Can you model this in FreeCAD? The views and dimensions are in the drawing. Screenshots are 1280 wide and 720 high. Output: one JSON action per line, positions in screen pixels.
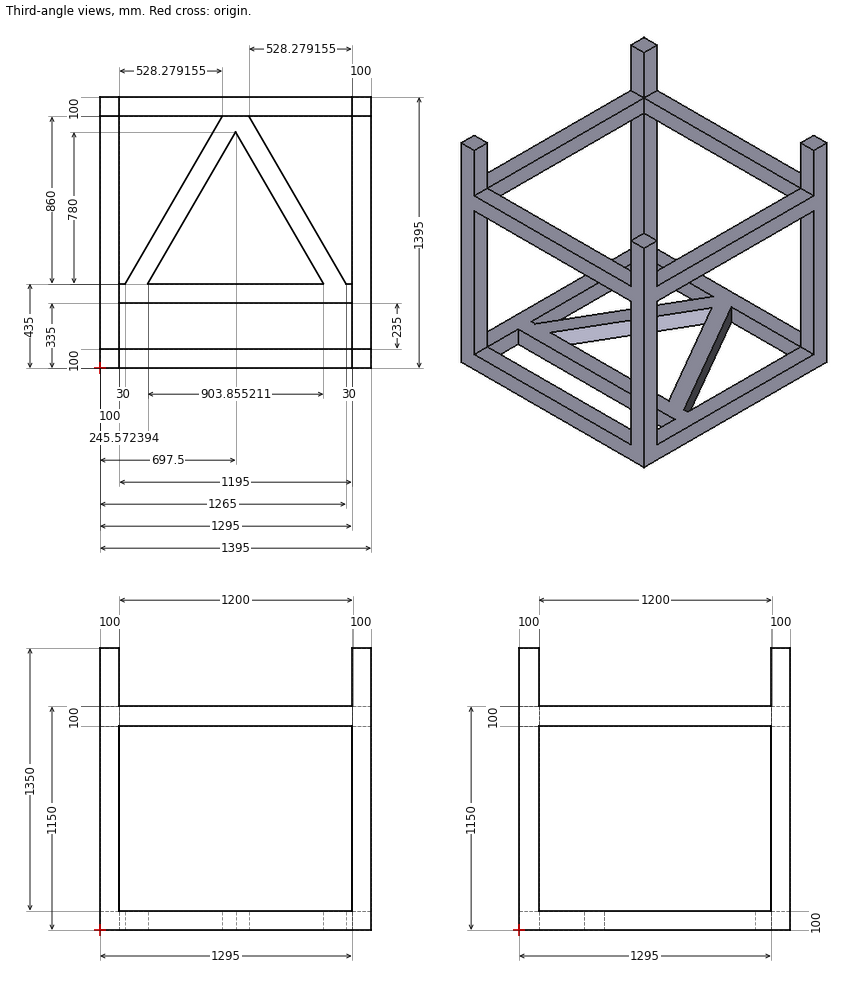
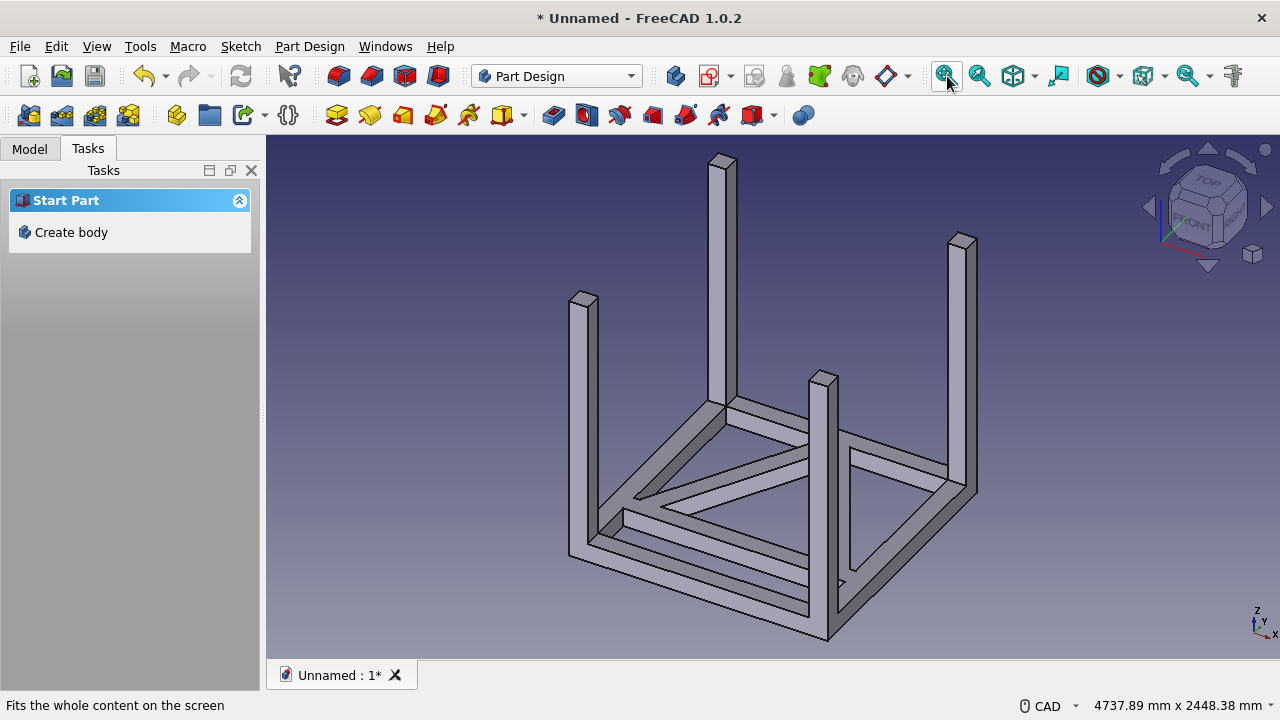
{"action": "left_click", "coordinate": [30, 148]}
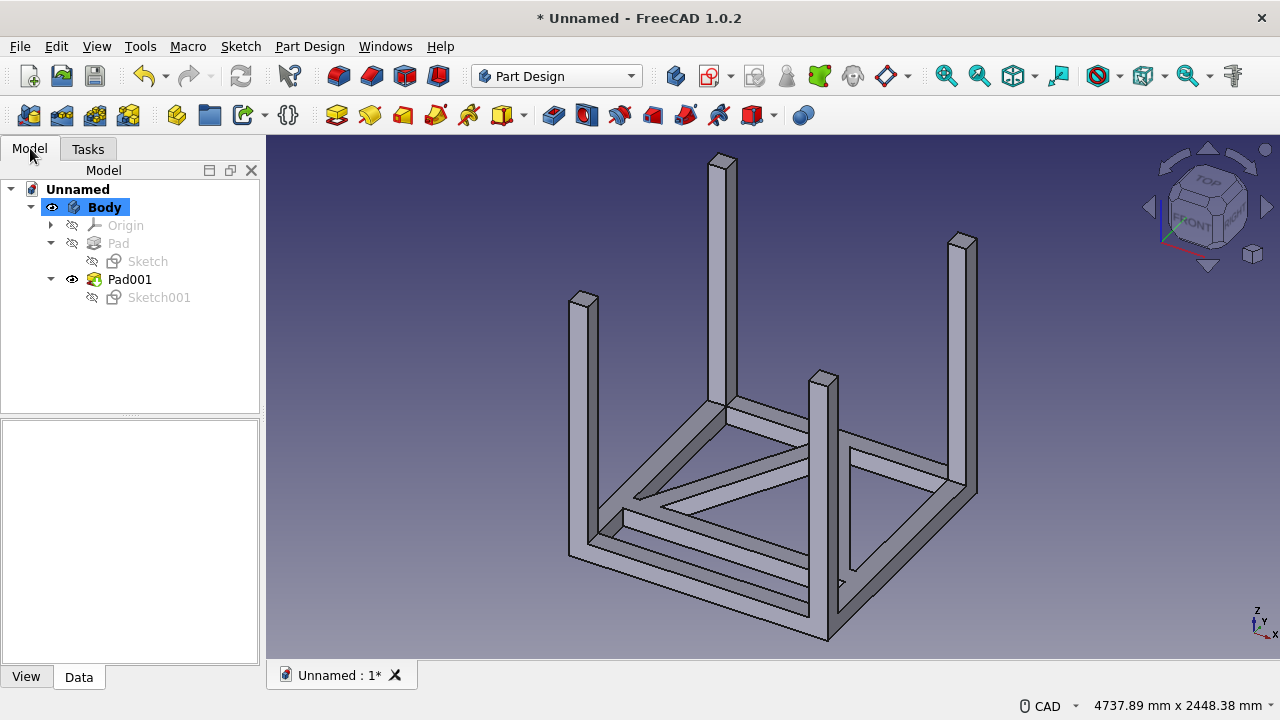
{"action": "left_click", "coordinate": [51, 225]}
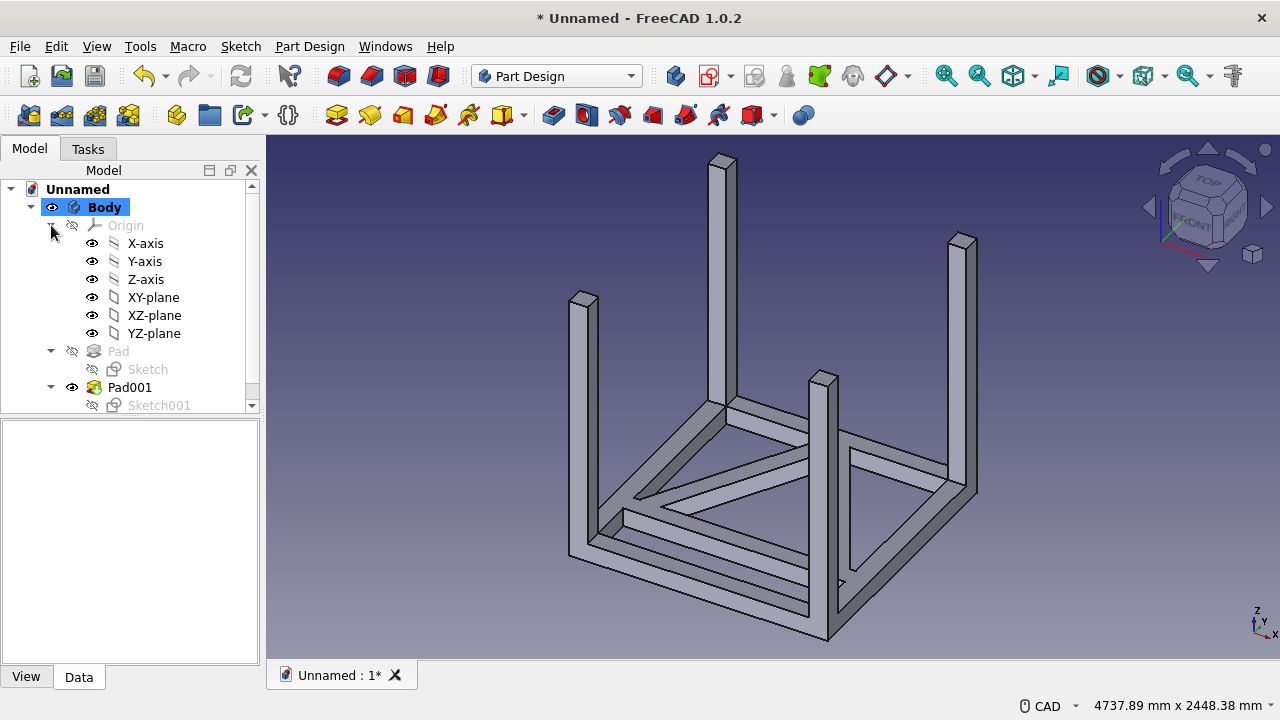
{"action": "left_click", "coordinate": [137, 333]}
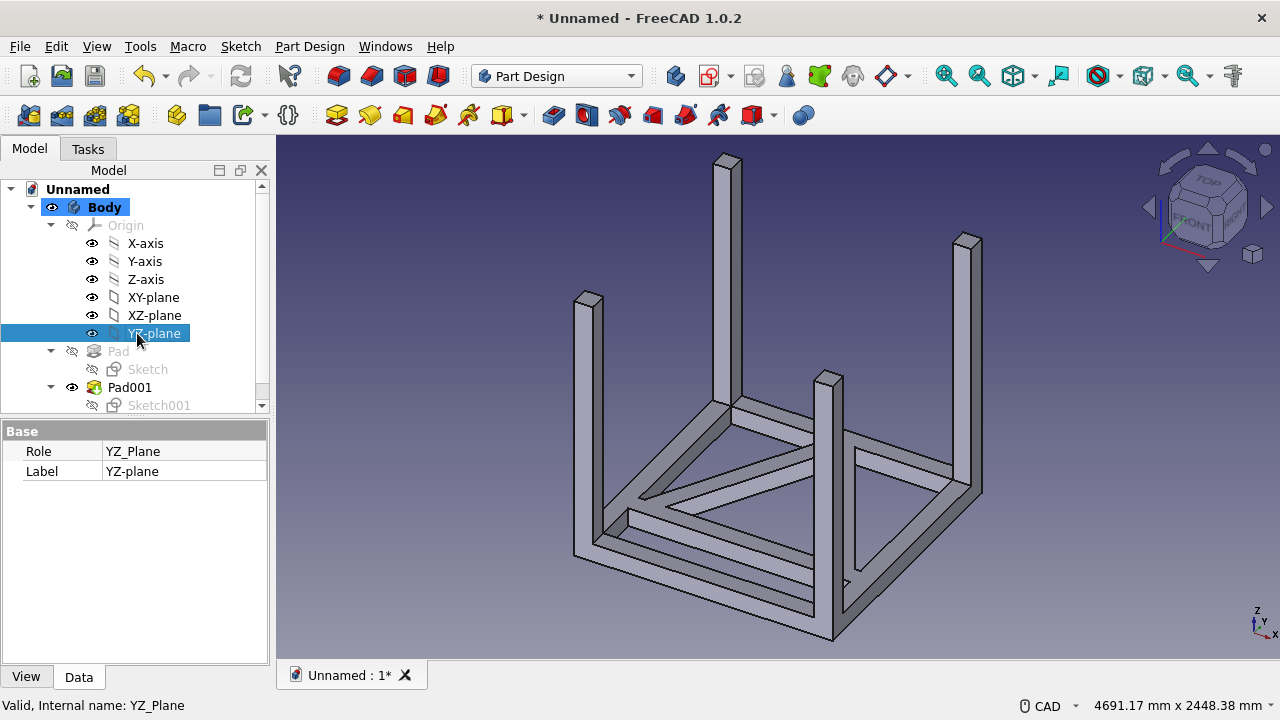
{"action": "left_click", "coordinate": [886, 76]}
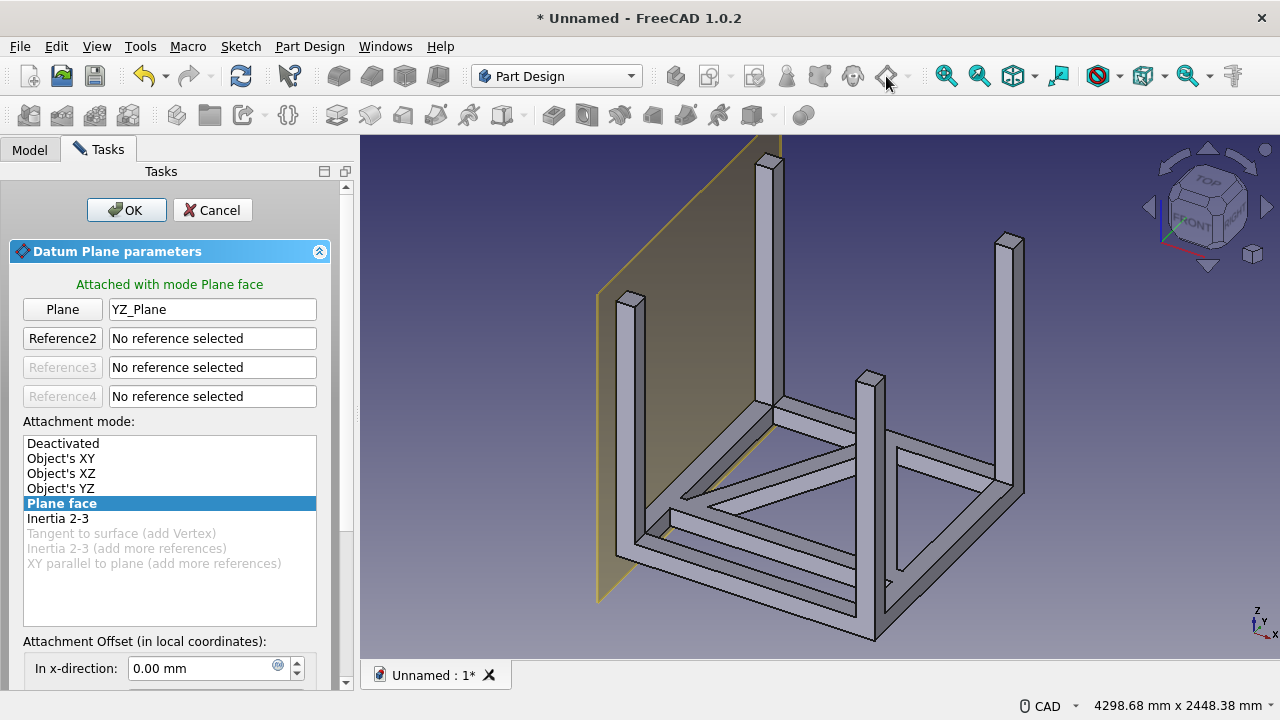
{"action": "scroll", "coordinate": [346, 436], "scroll_direction": "down", "scroll_amount": 2}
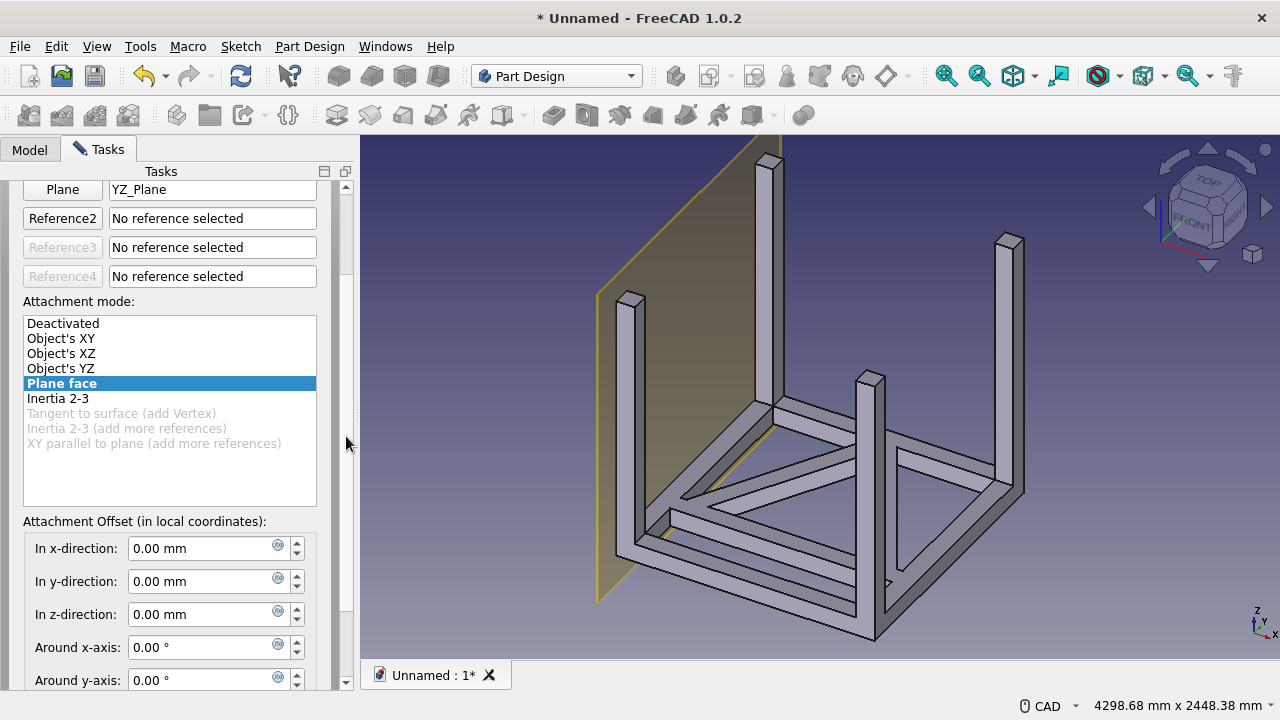
{"action": "triple_click", "coordinate": [210, 614]}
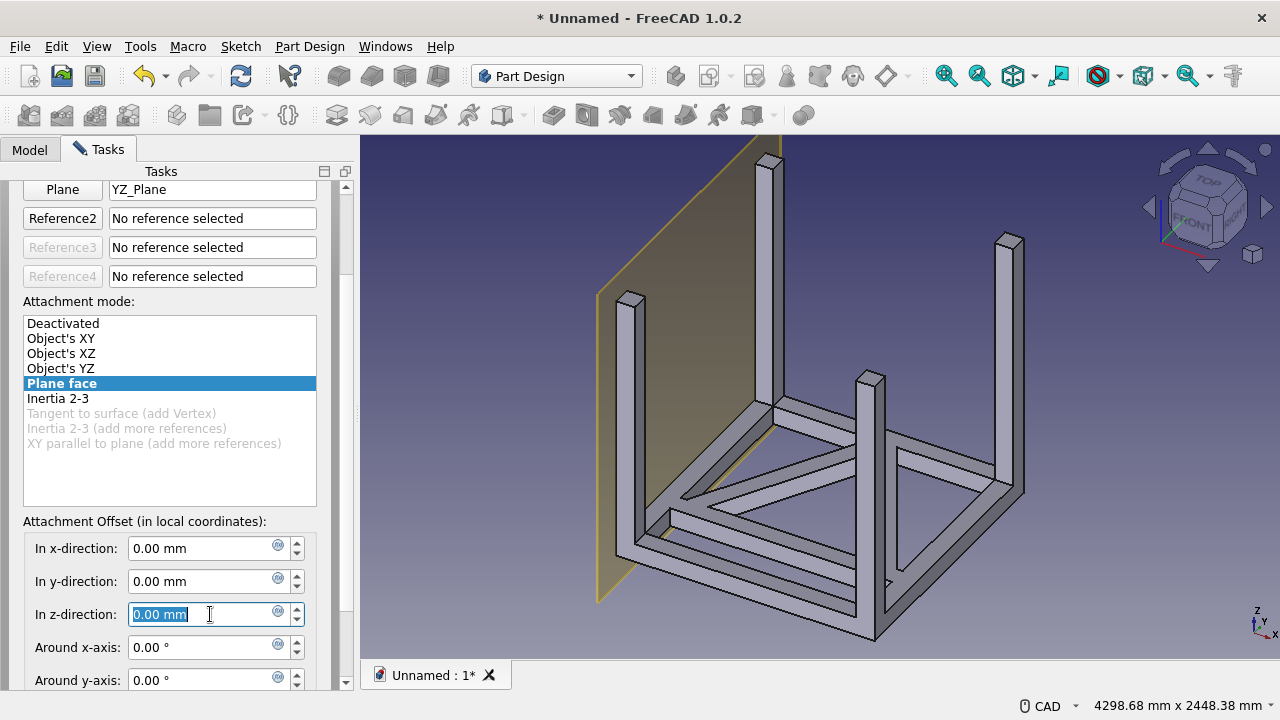
{"action": "type", "text": "100"}
{"action": "key", "text": "Tab"}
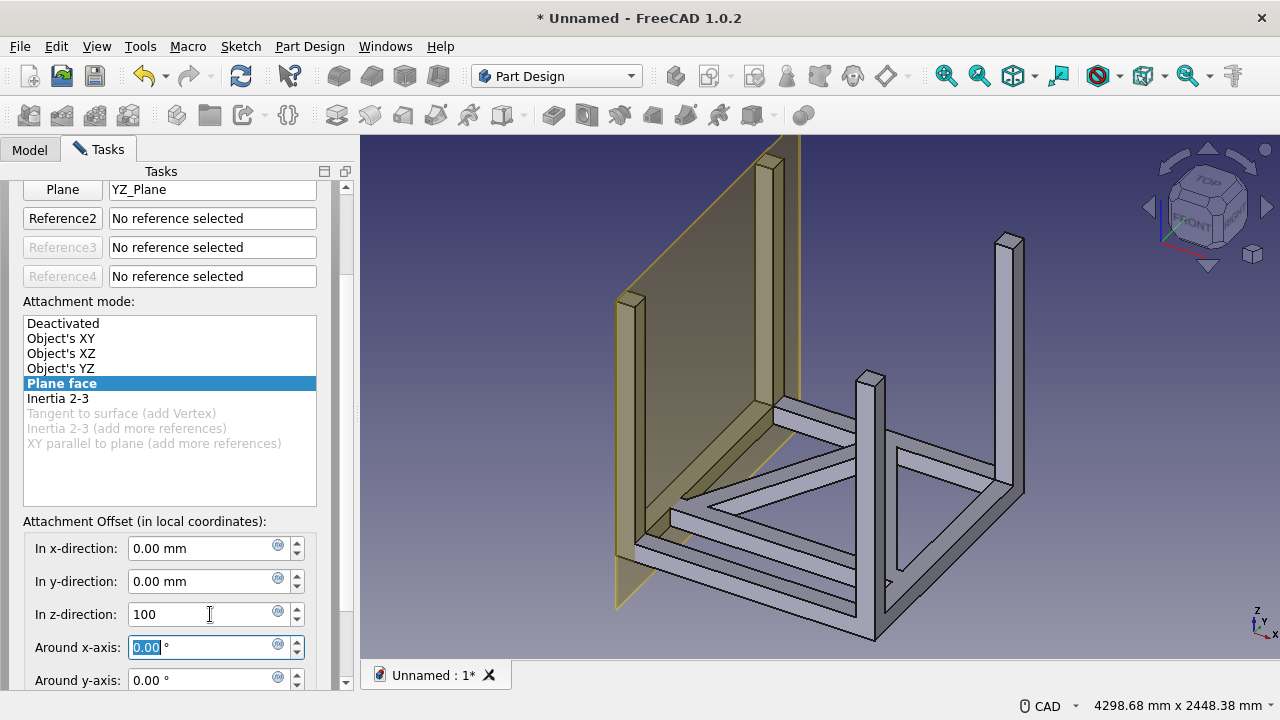
{"action": "scroll", "coordinate": [346, 436], "scroll_direction": "up", "scroll_amount": 3}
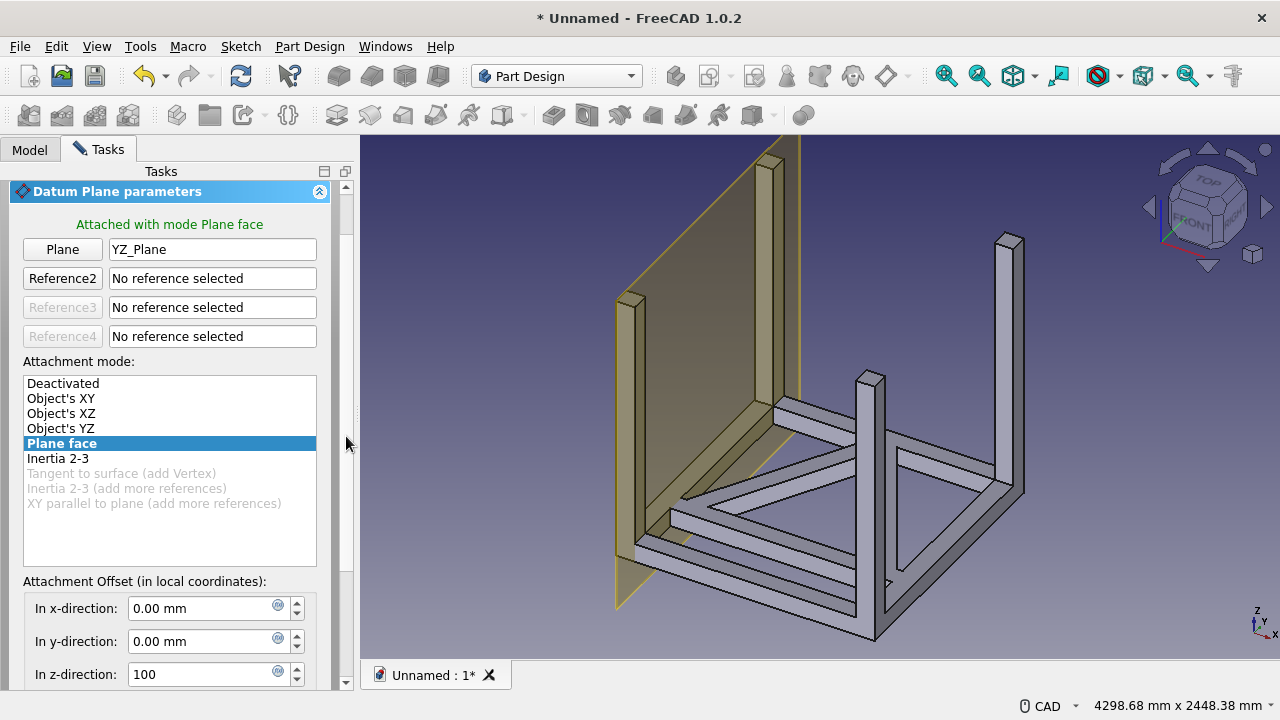
{"action": "left_click", "coordinate": [127, 210]}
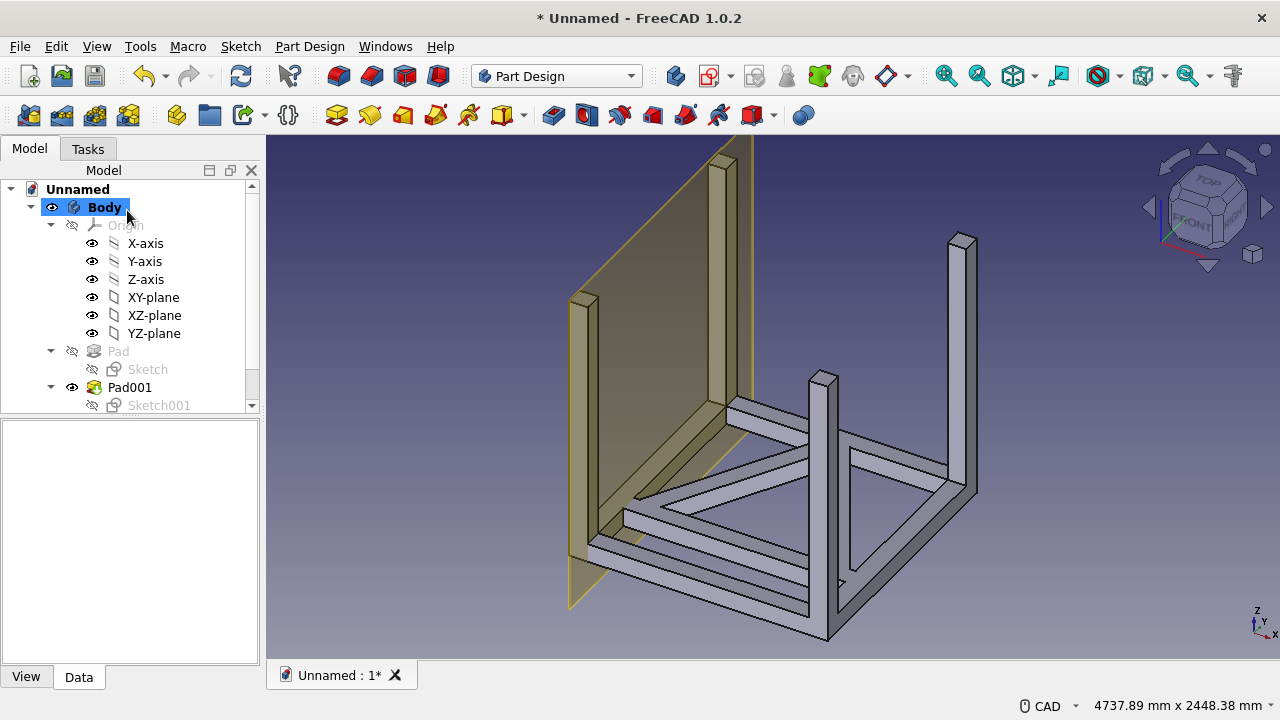
{"action": "scroll", "coordinate": [101, 293], "scroll_direction": "down", "scroll_amount": 3}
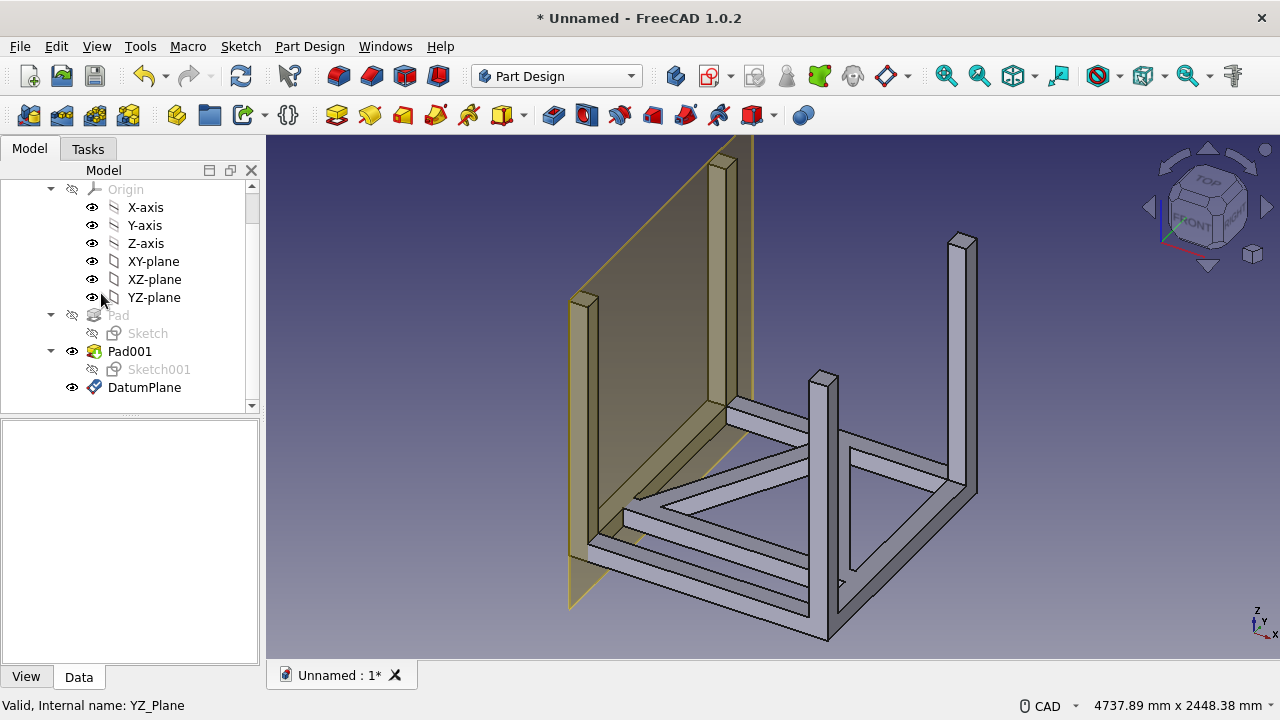
{"action": "left_click", "coordinate": [117, 387]}